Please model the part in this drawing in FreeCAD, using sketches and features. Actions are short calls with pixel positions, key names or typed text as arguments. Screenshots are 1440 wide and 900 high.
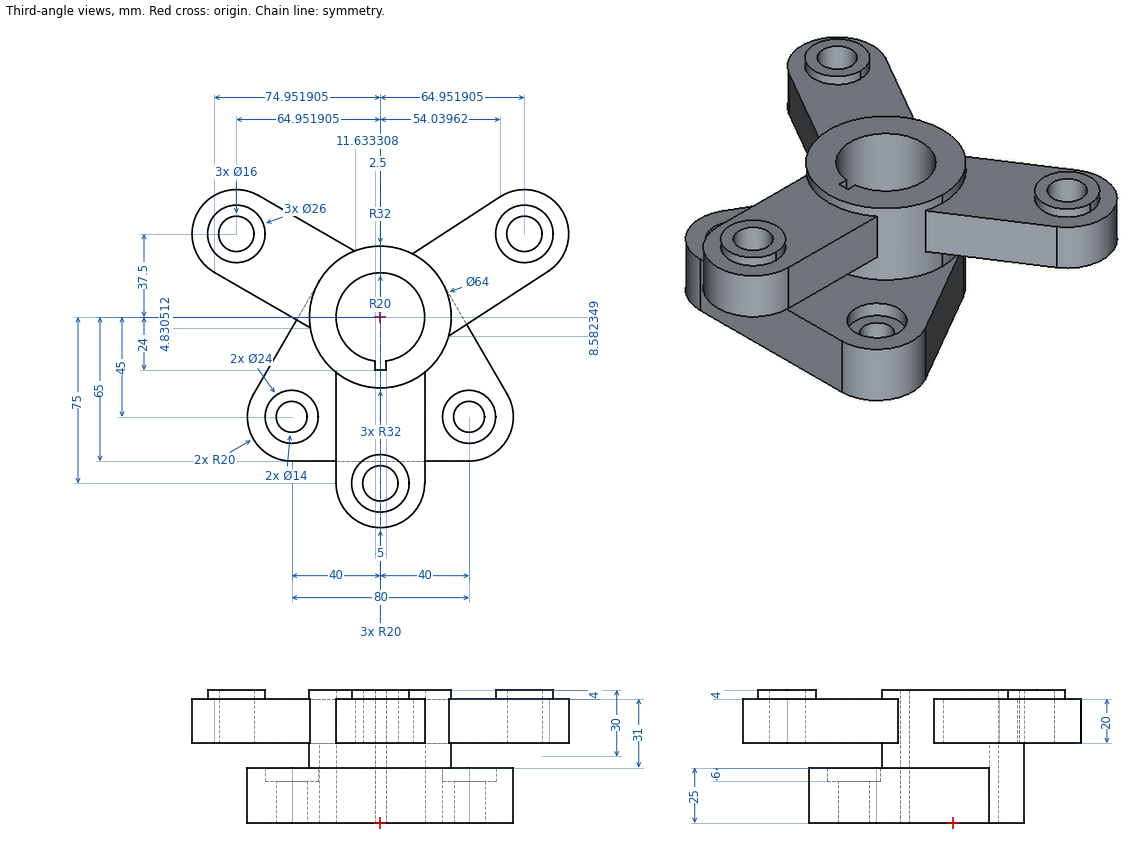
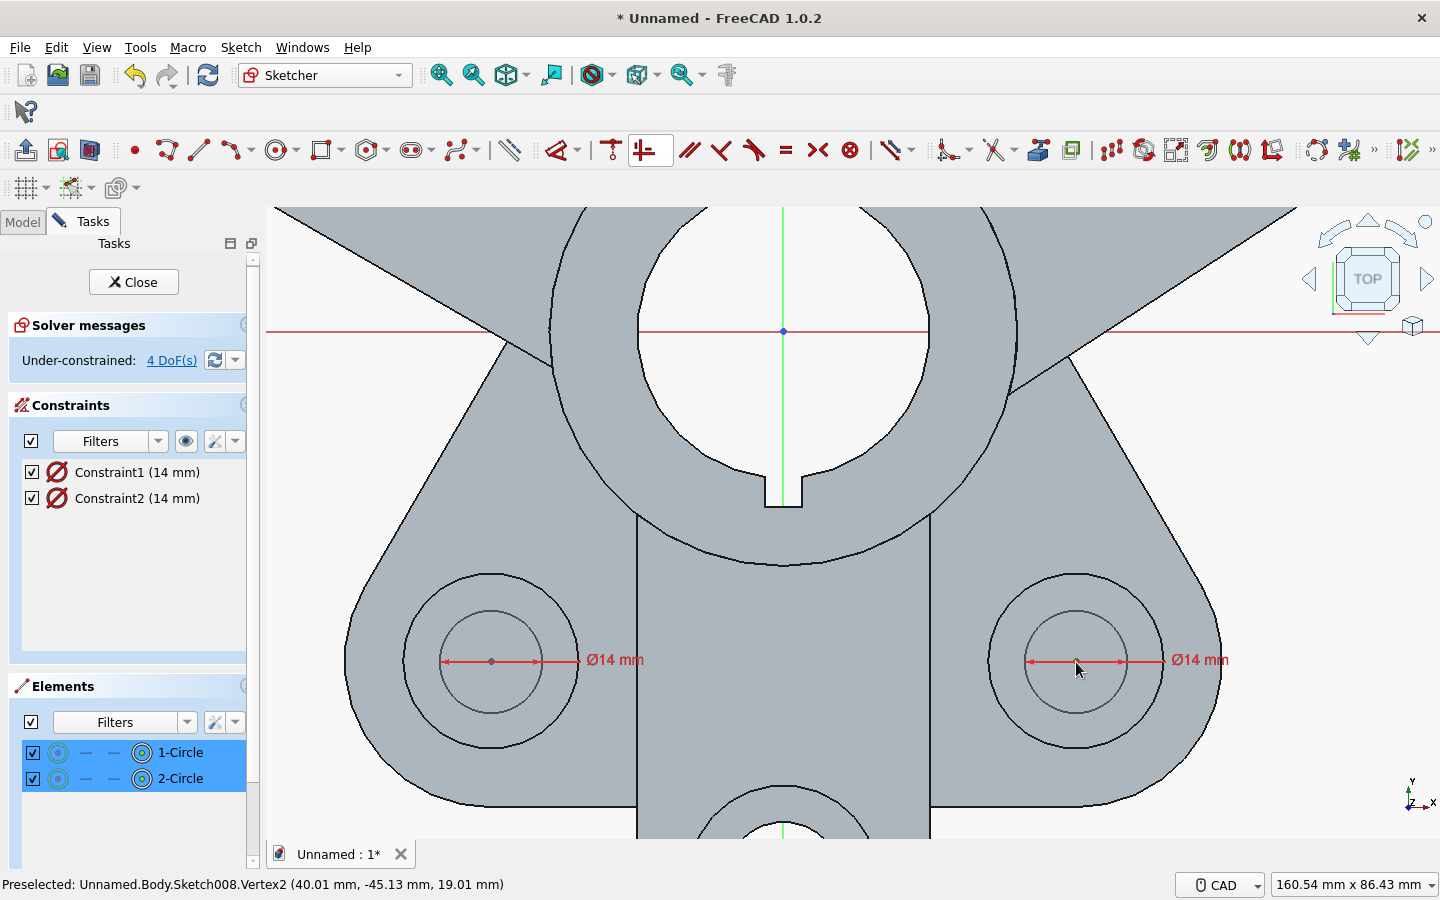
key(h)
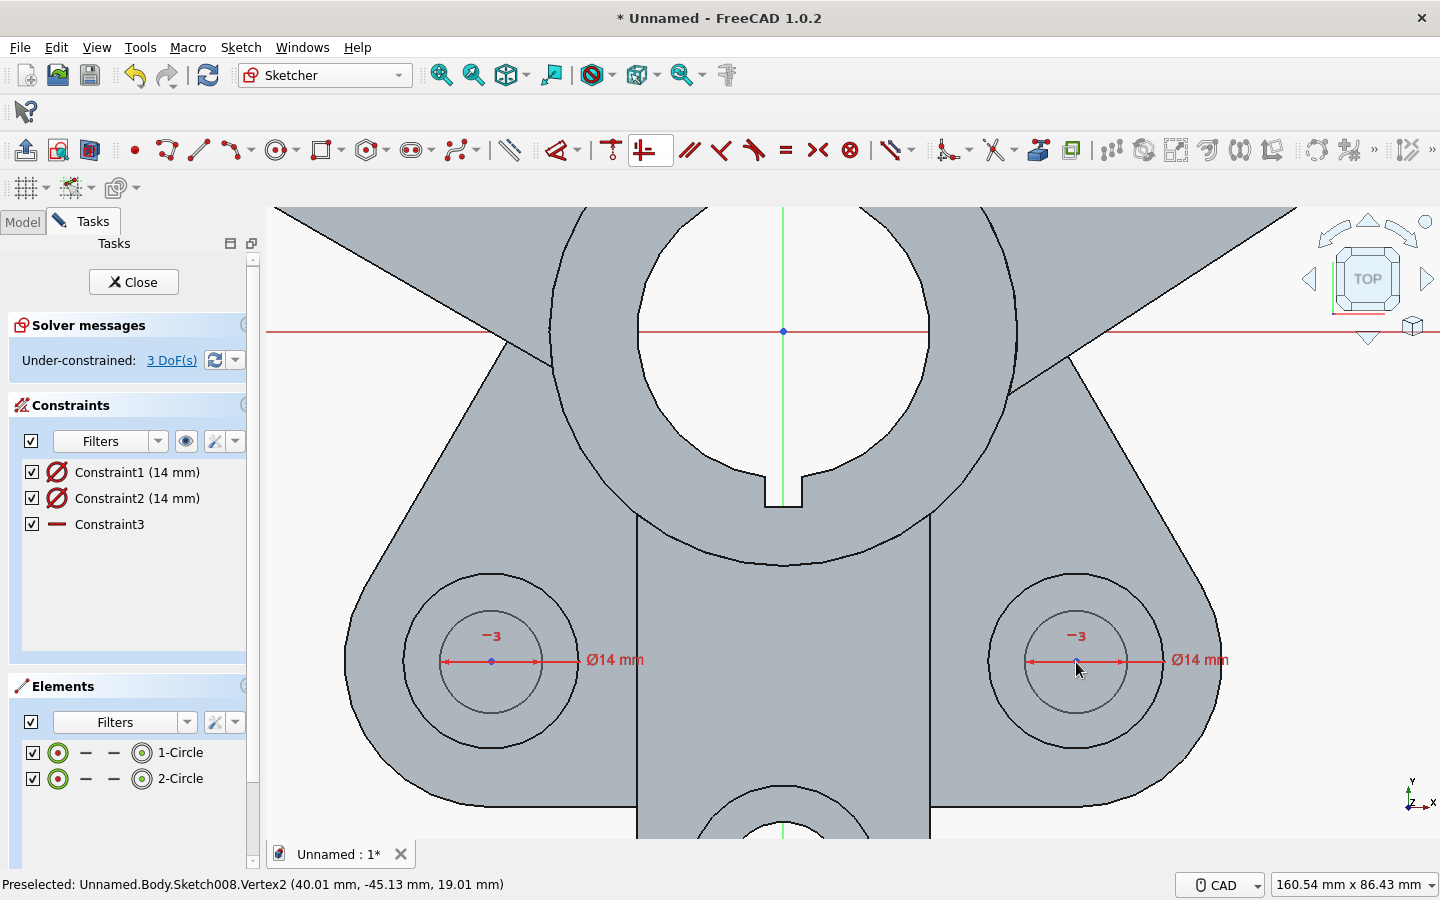
click(556, 150)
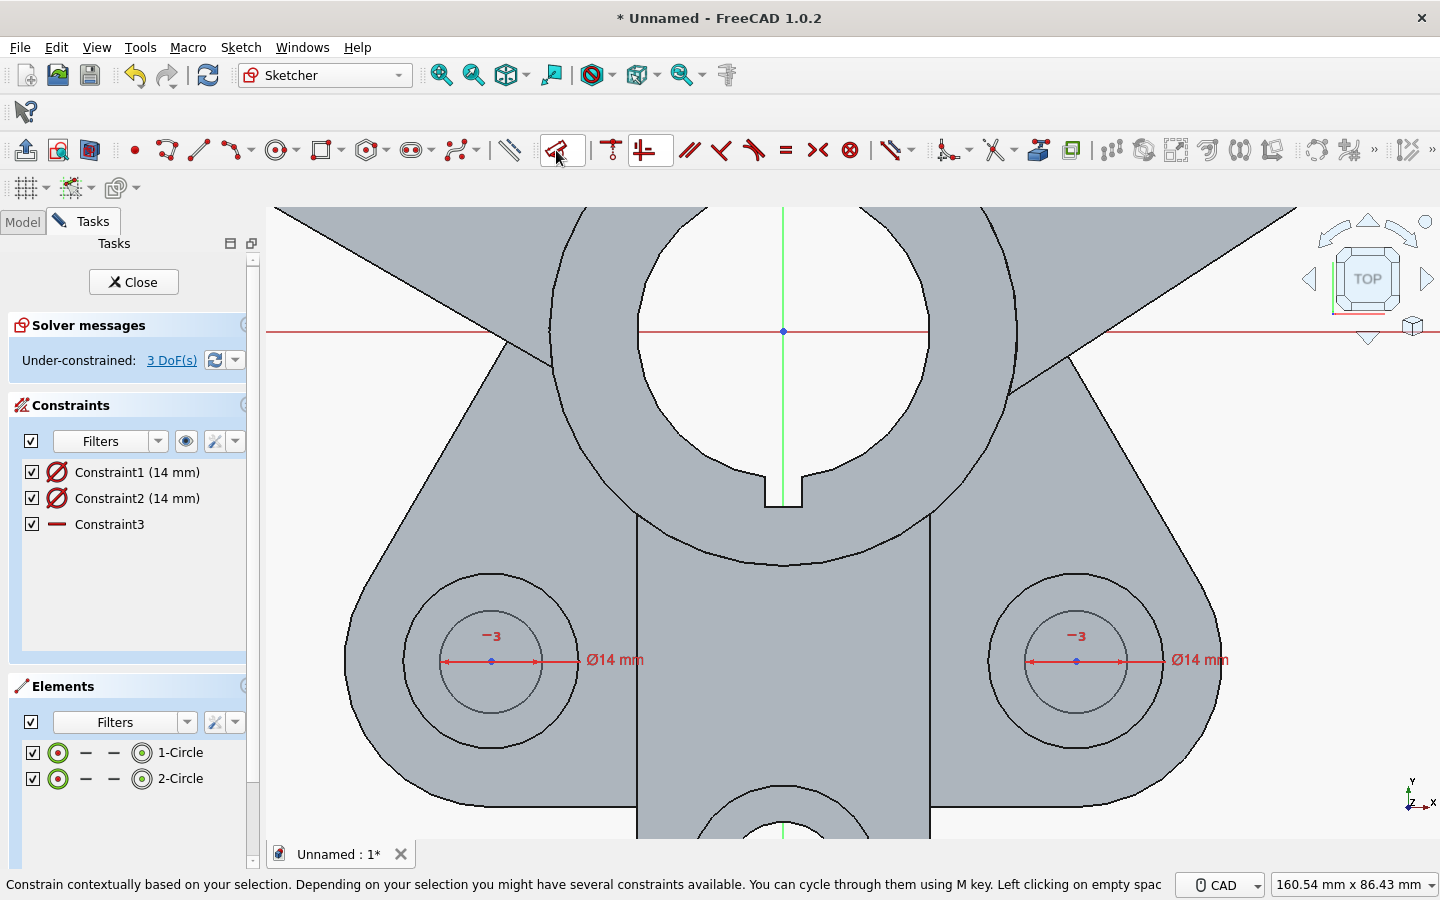
click(491, 662)
click(637, 298)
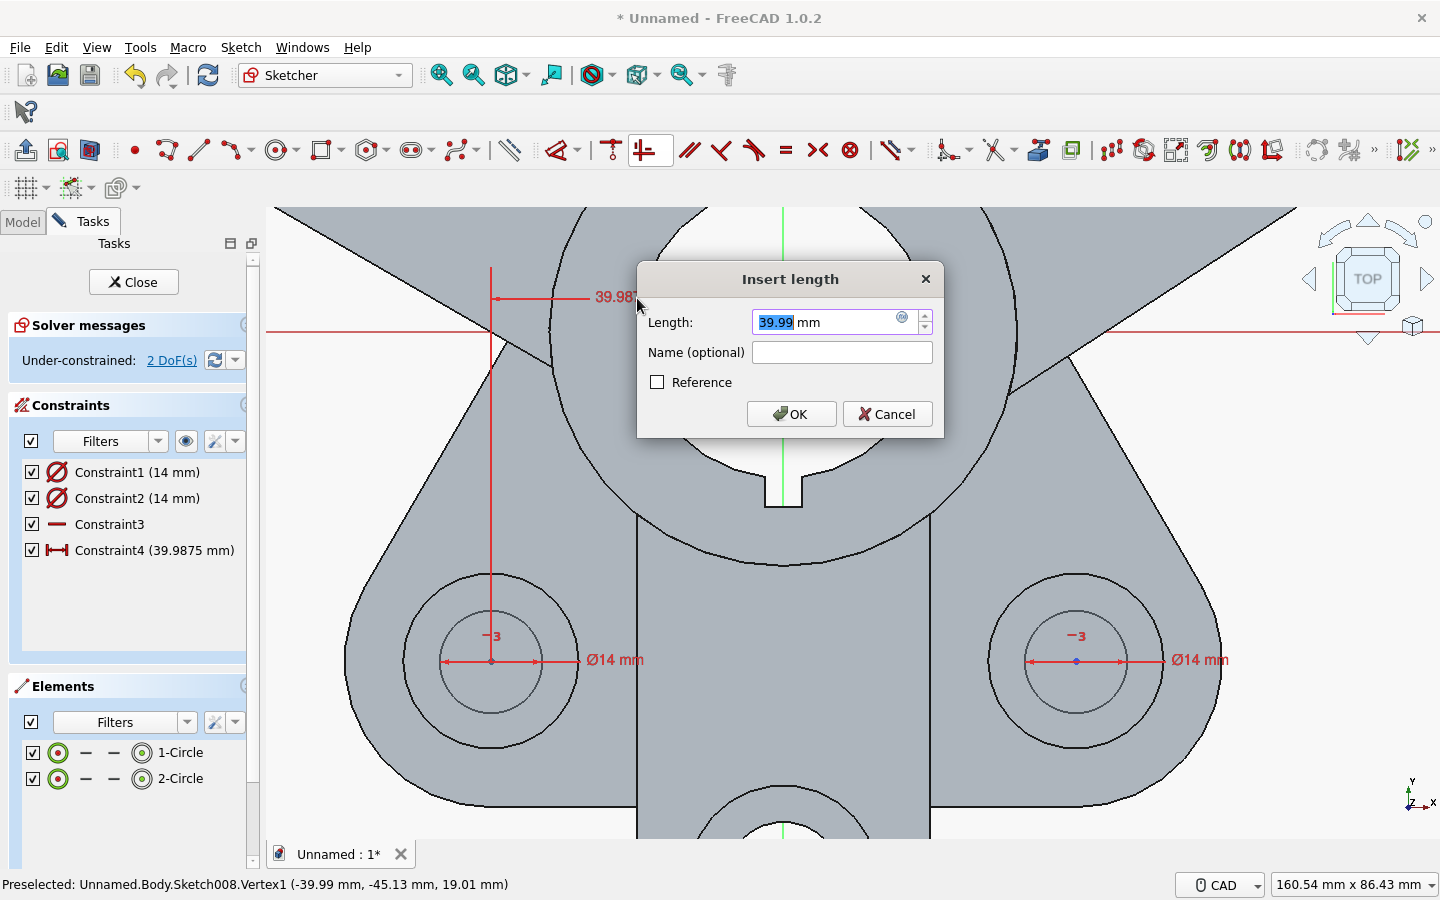
text(40)
key(Return)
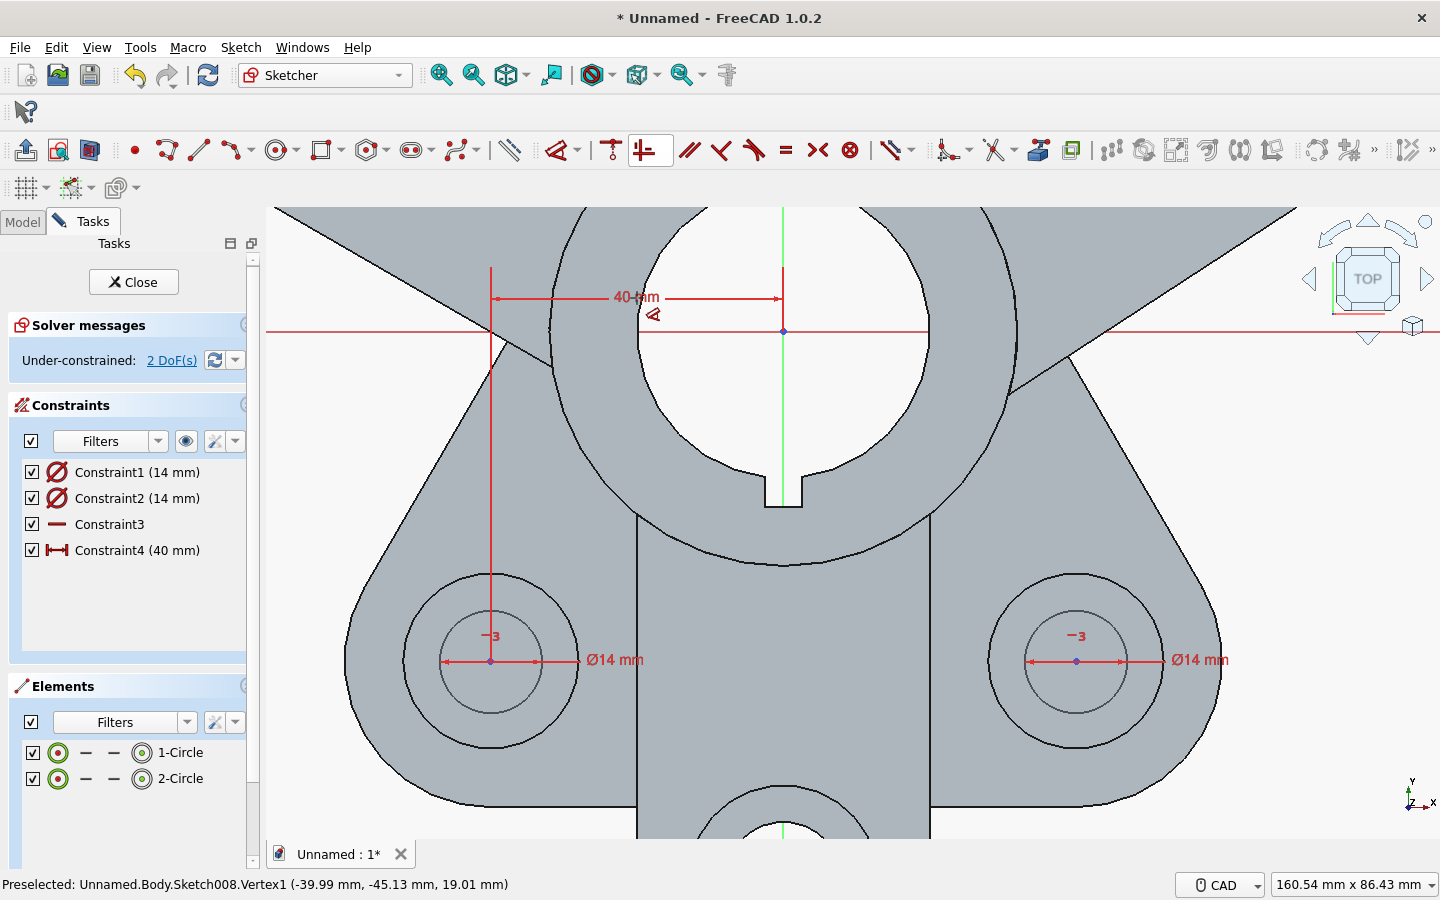
click(491, 662)
click(457, 497)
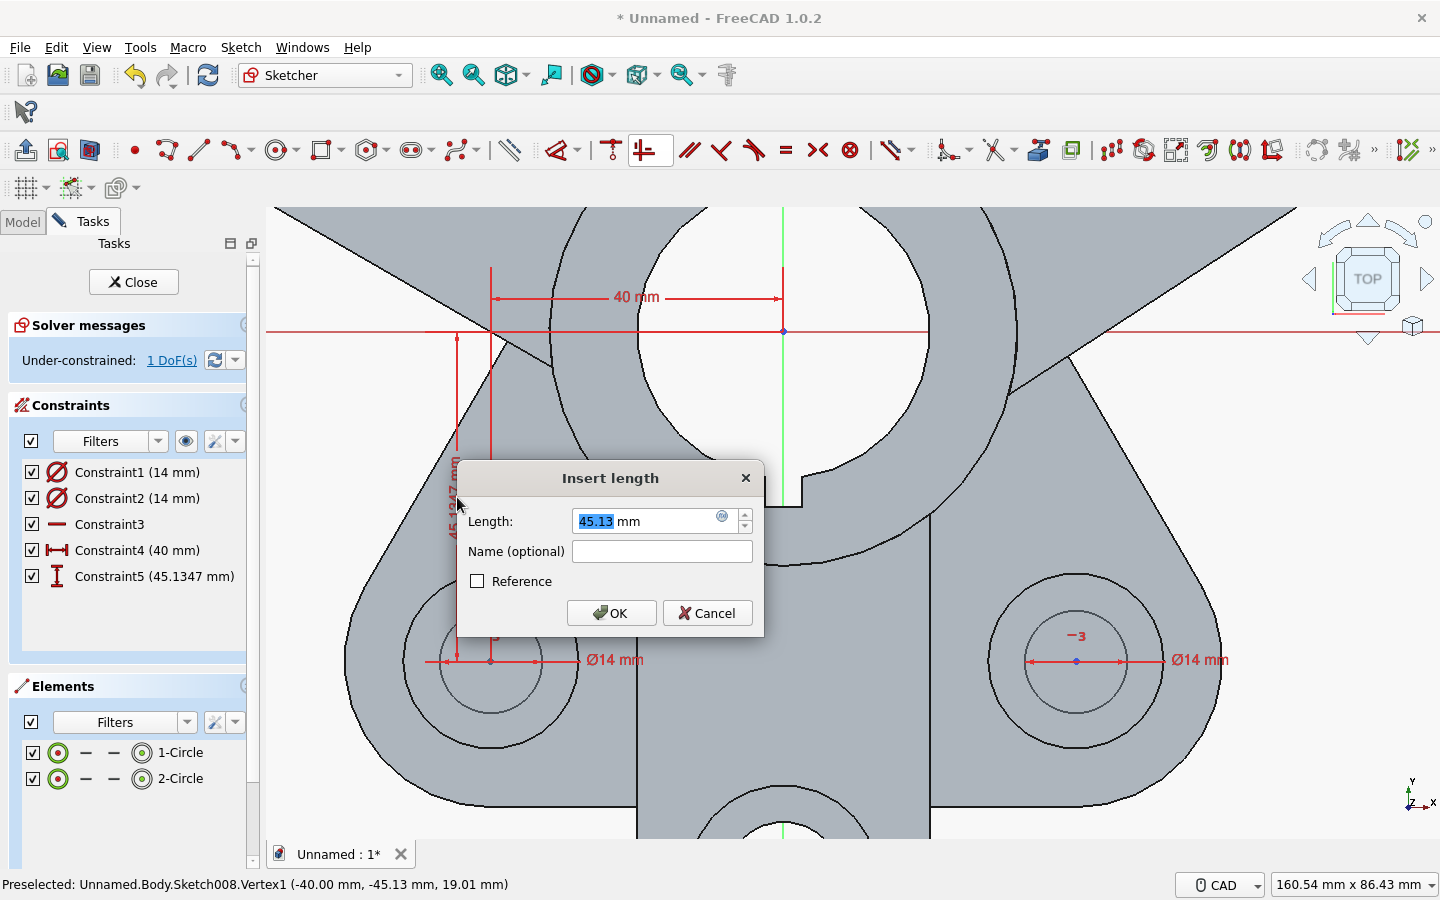
text(45)
key(Return)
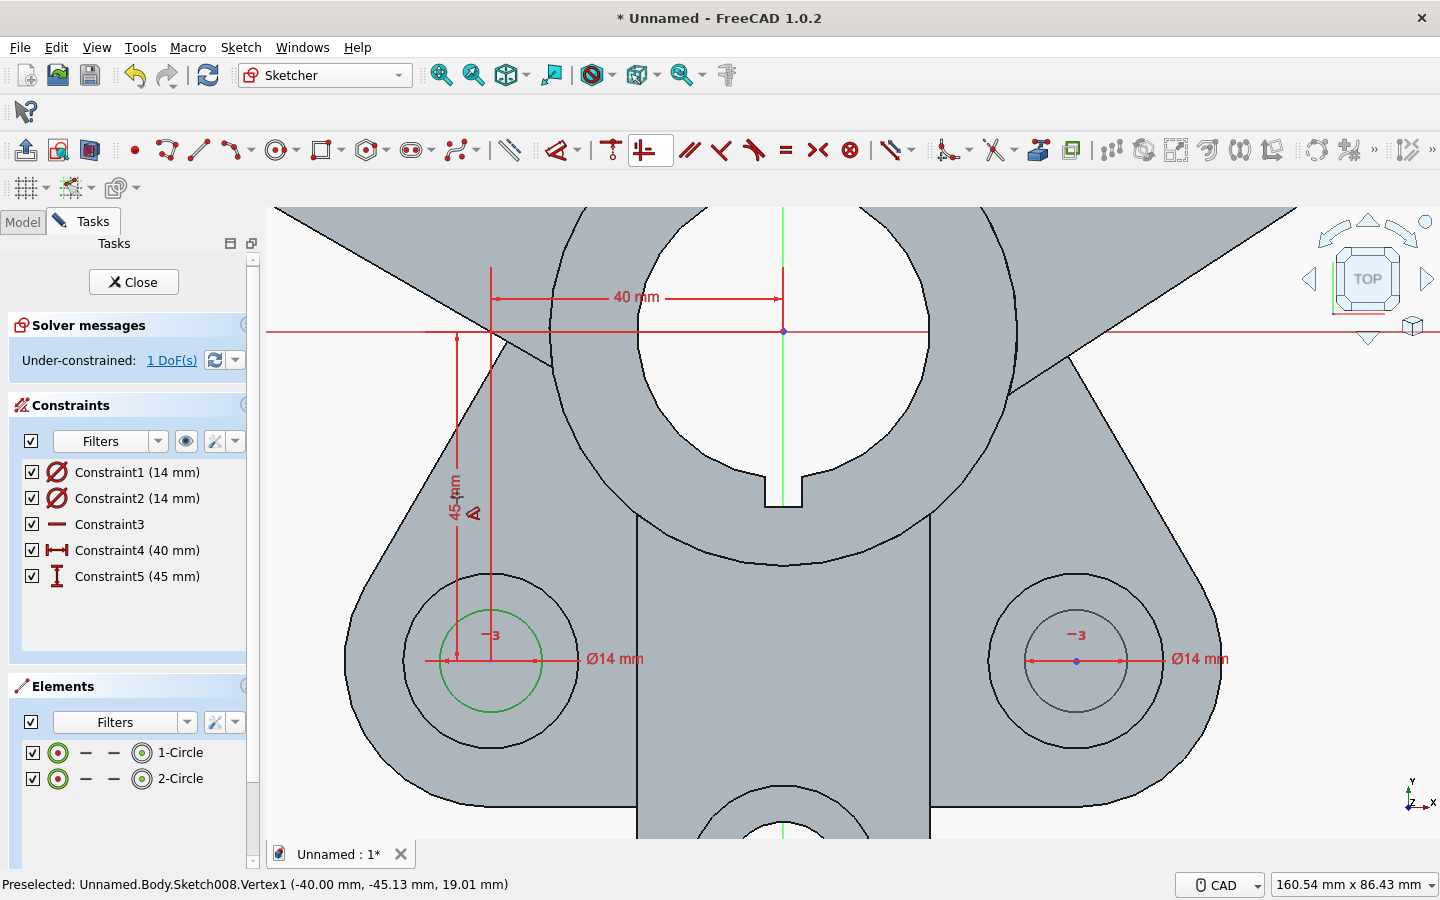
click(1076, 661)
click(930, 298)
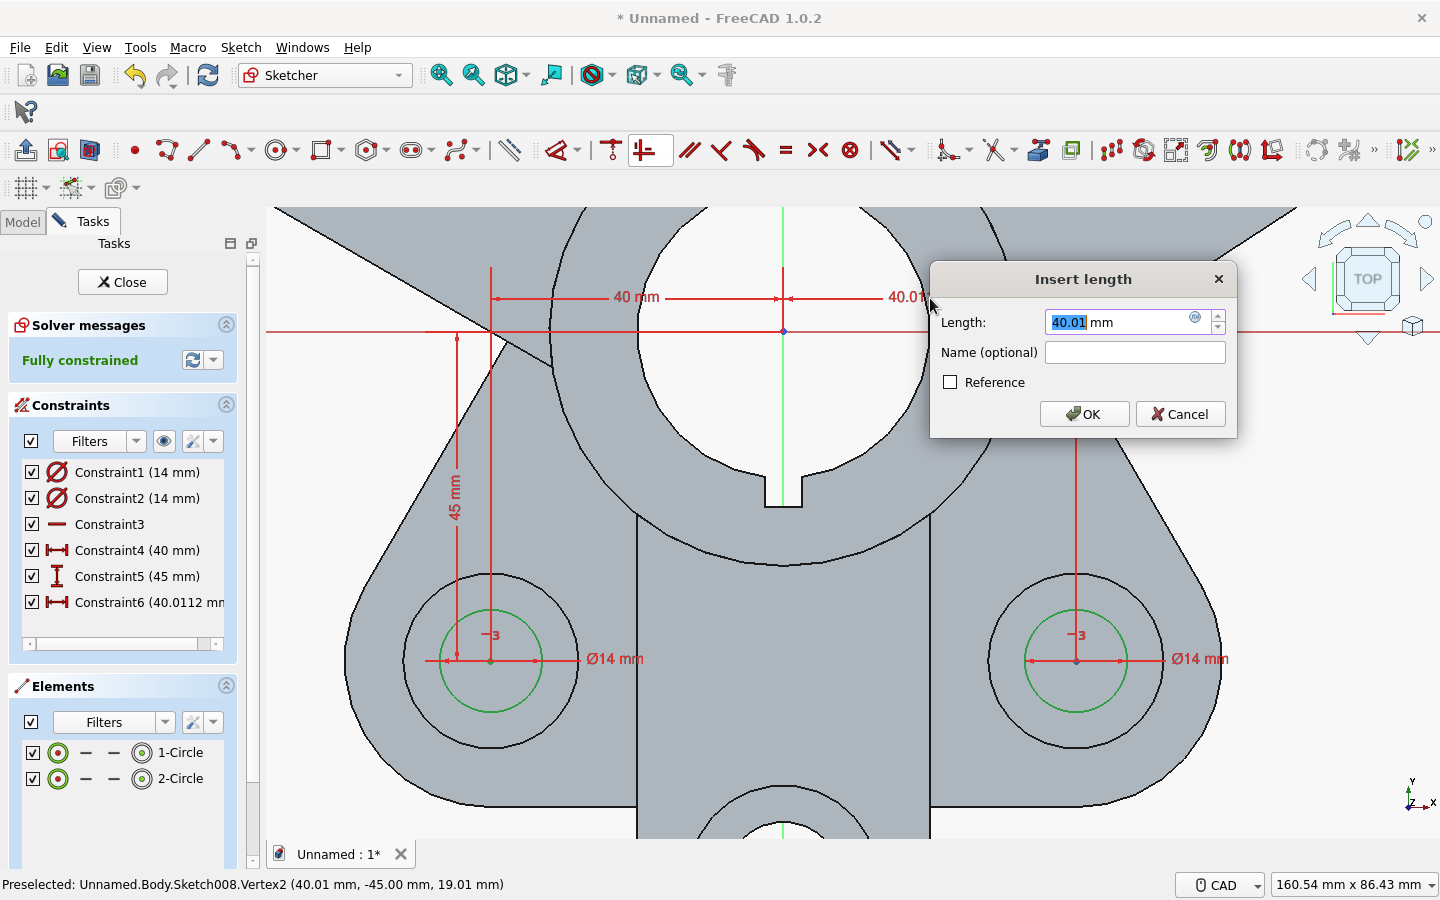
text(40)
key(Return)
key(Escape)